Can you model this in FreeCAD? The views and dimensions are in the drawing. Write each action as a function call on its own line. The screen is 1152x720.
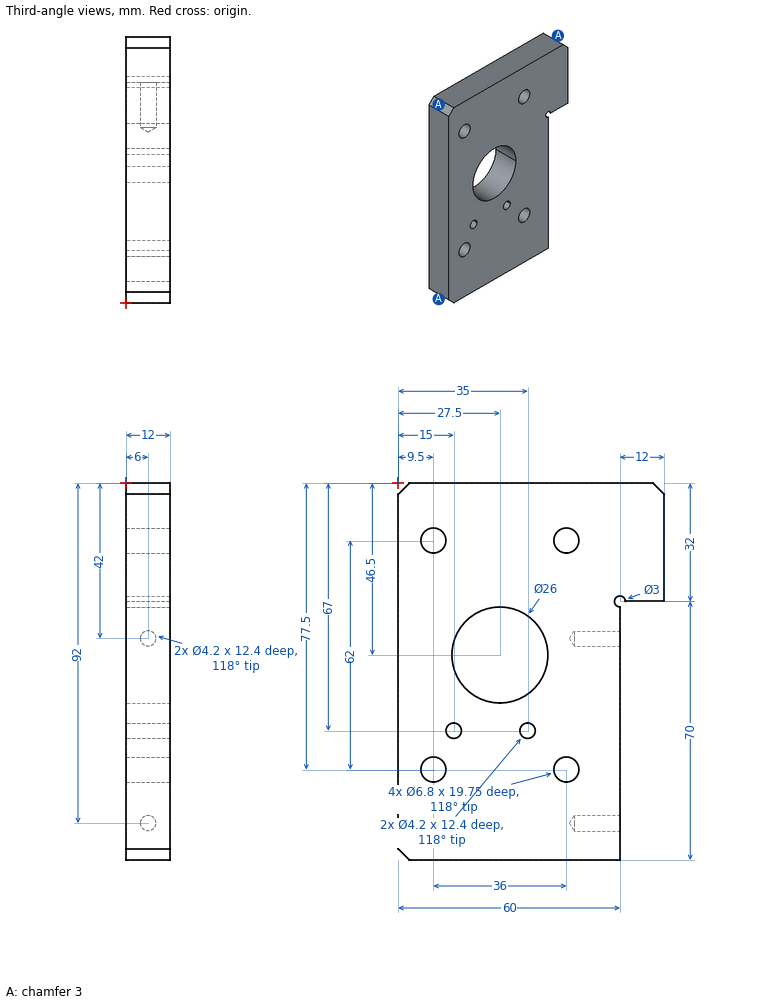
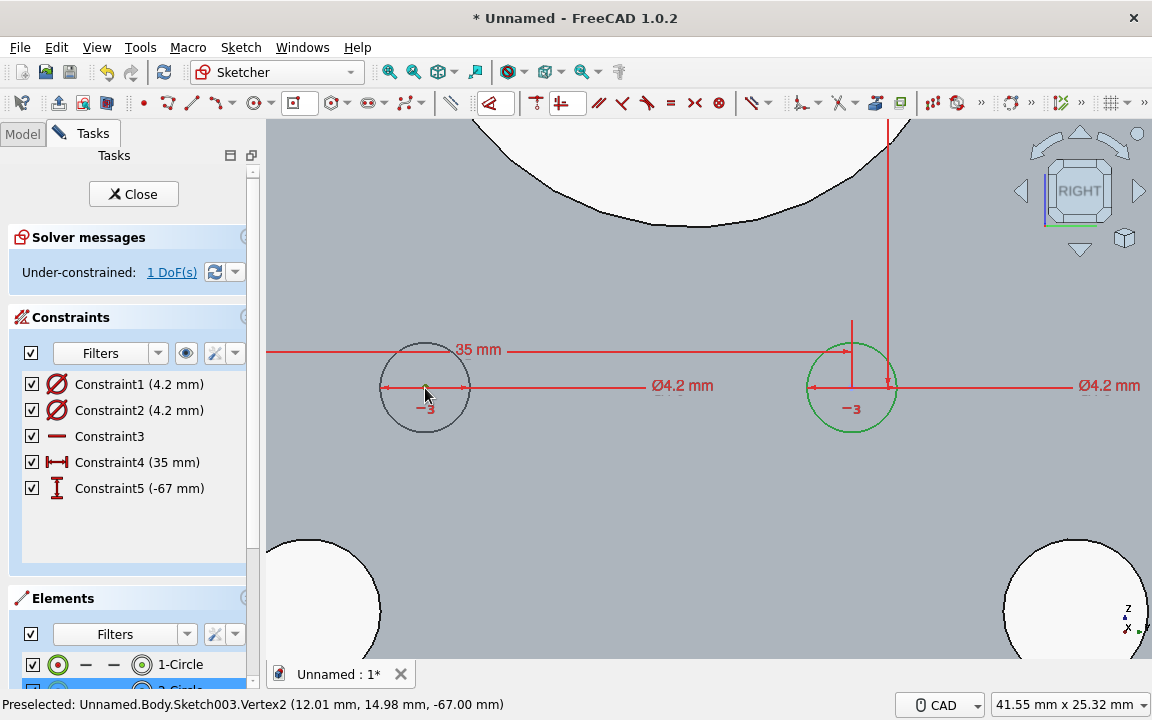
key(l)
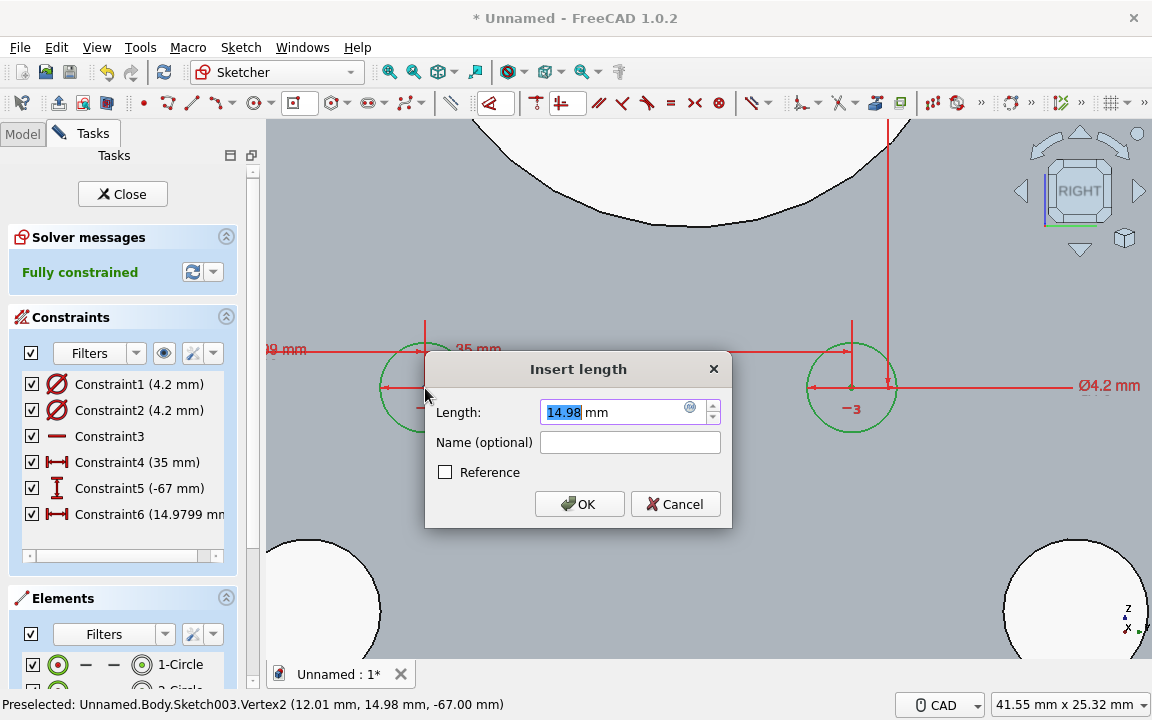
text(15)
key(Return)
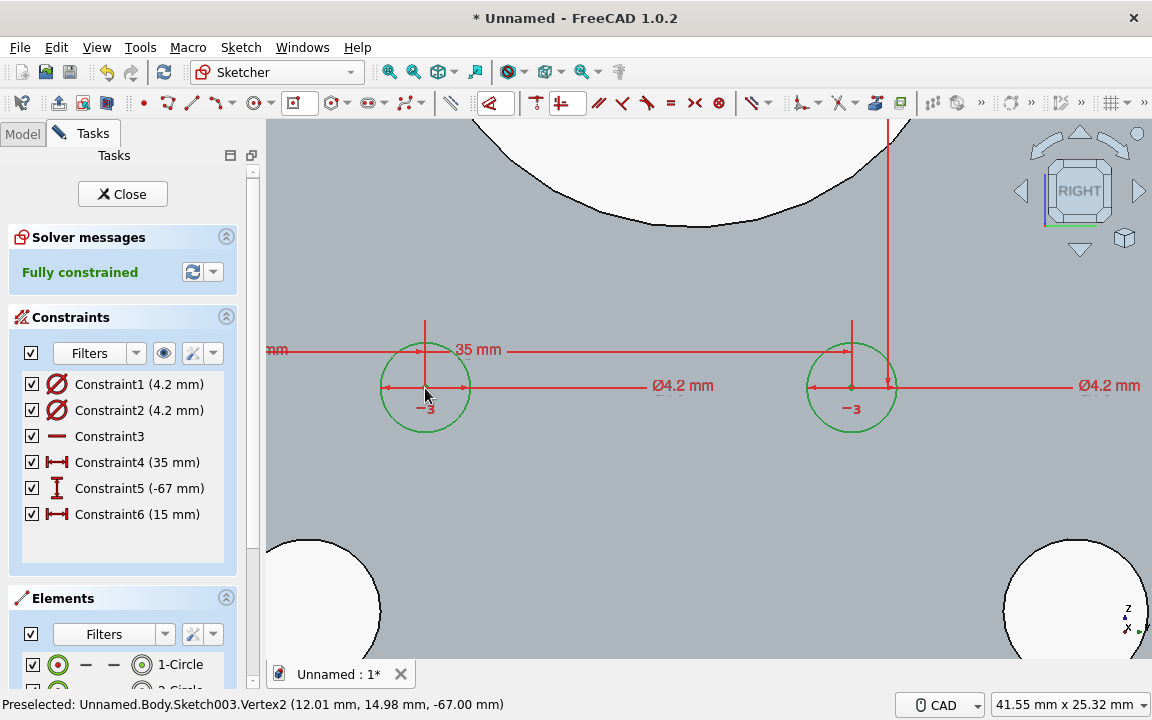
click(123, 194)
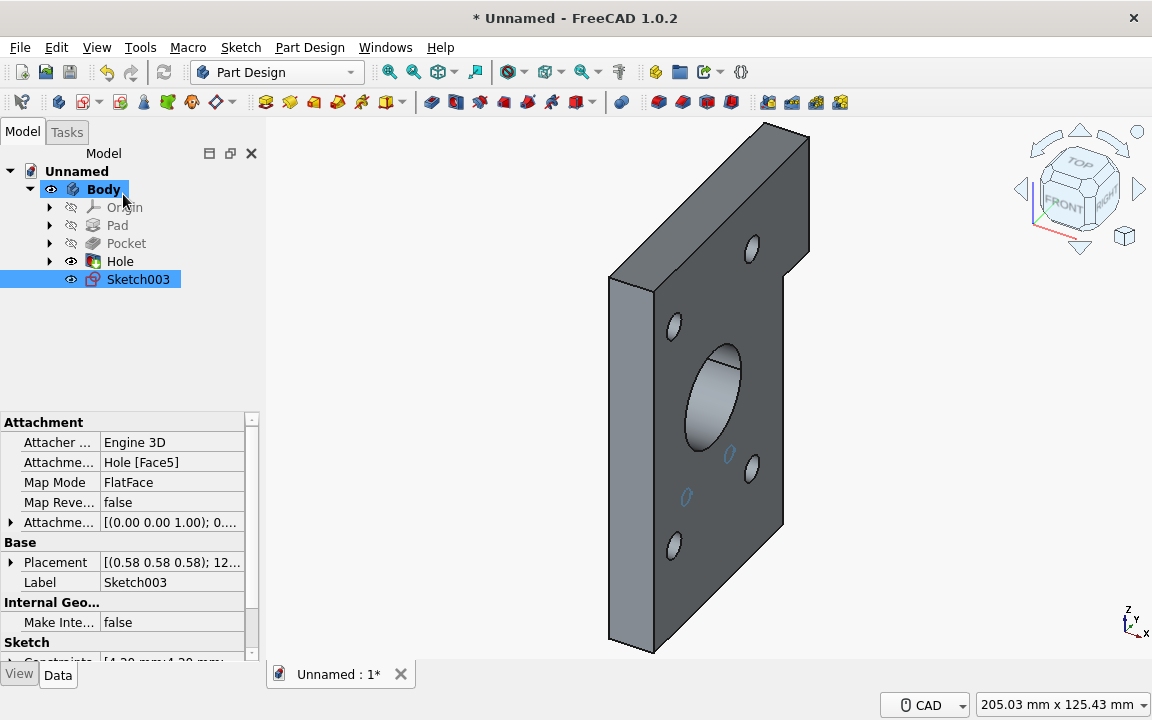
click(456, 102)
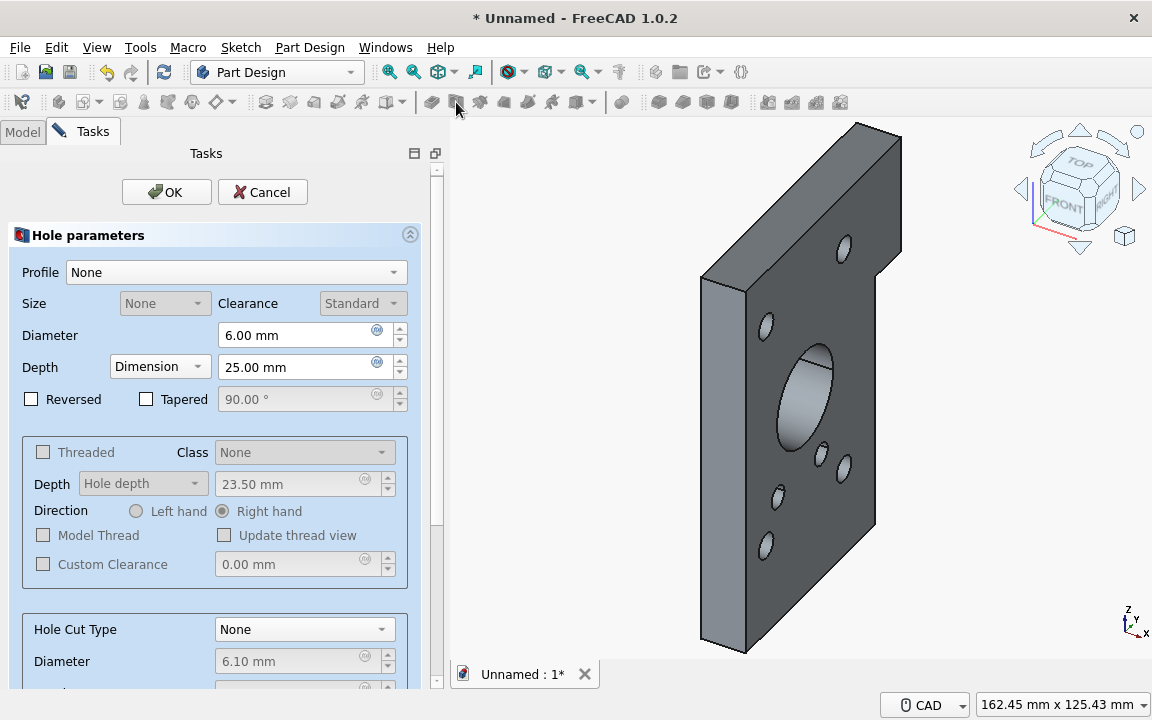
triple_click(305, 335)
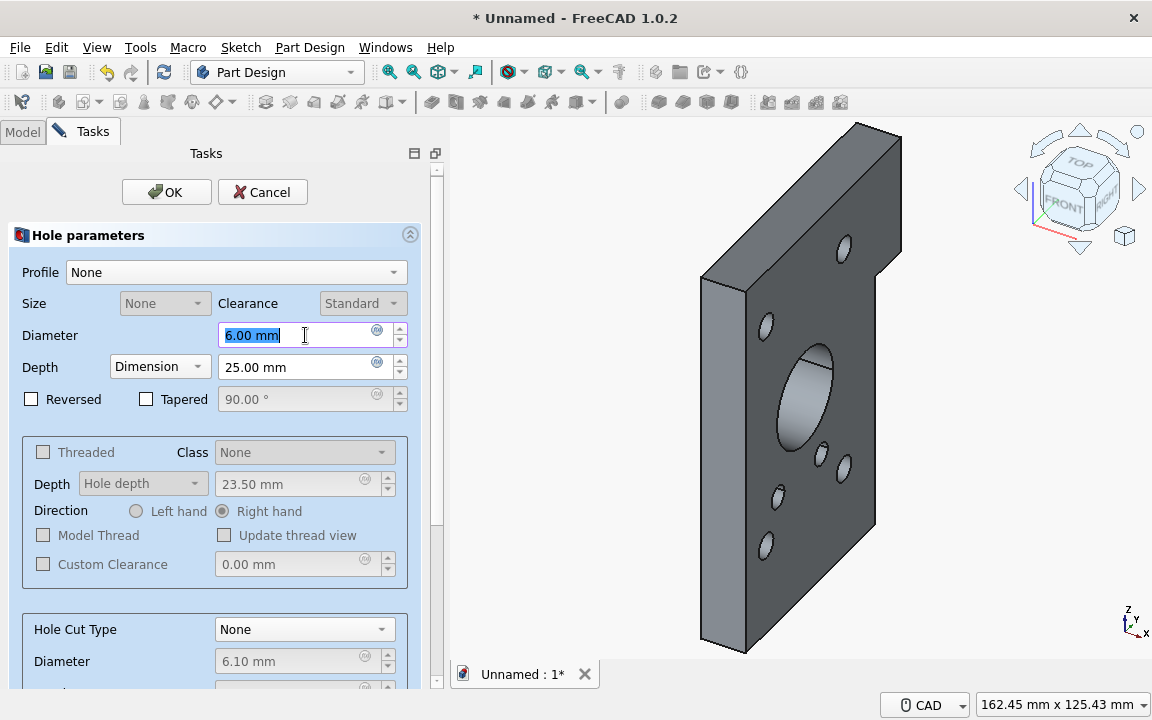
text(4.2)
key(Tab)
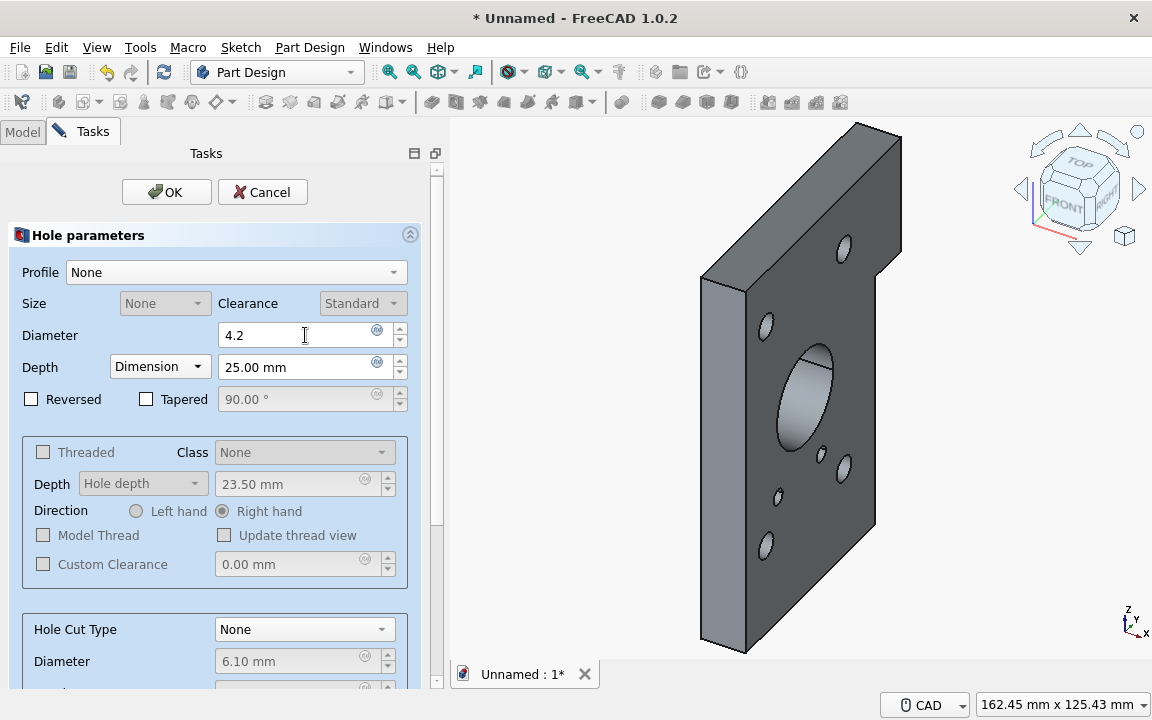
triple_click(305, 367)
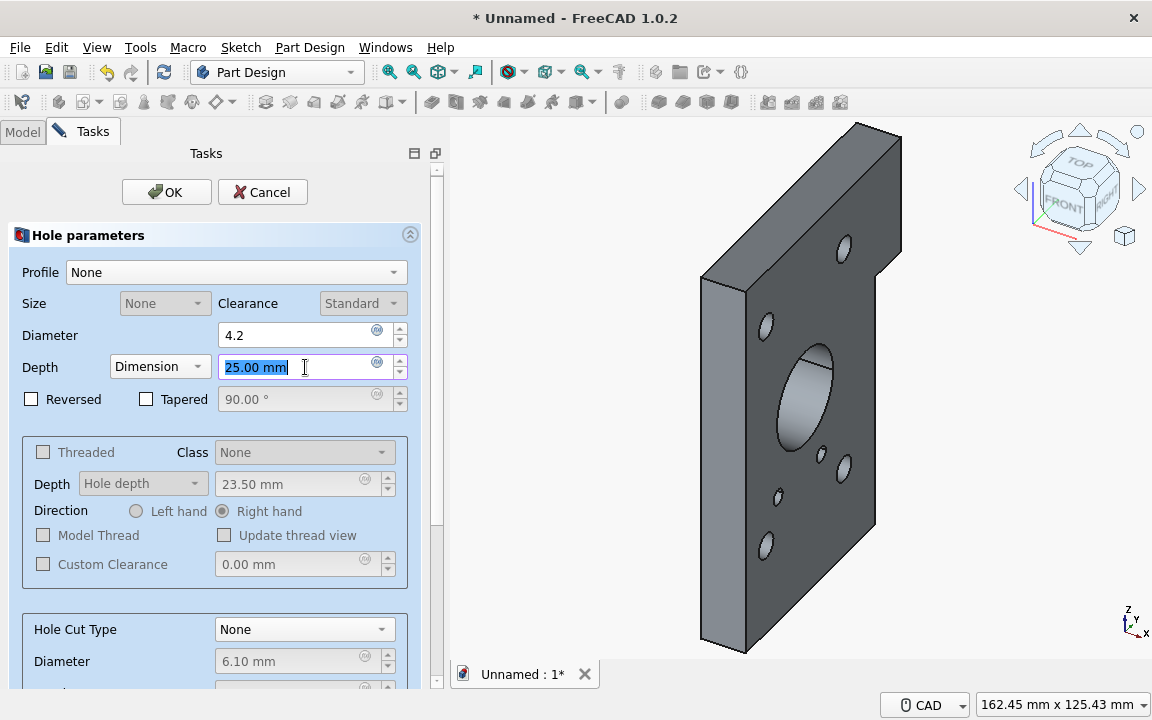
text(12.4)
key(Tab)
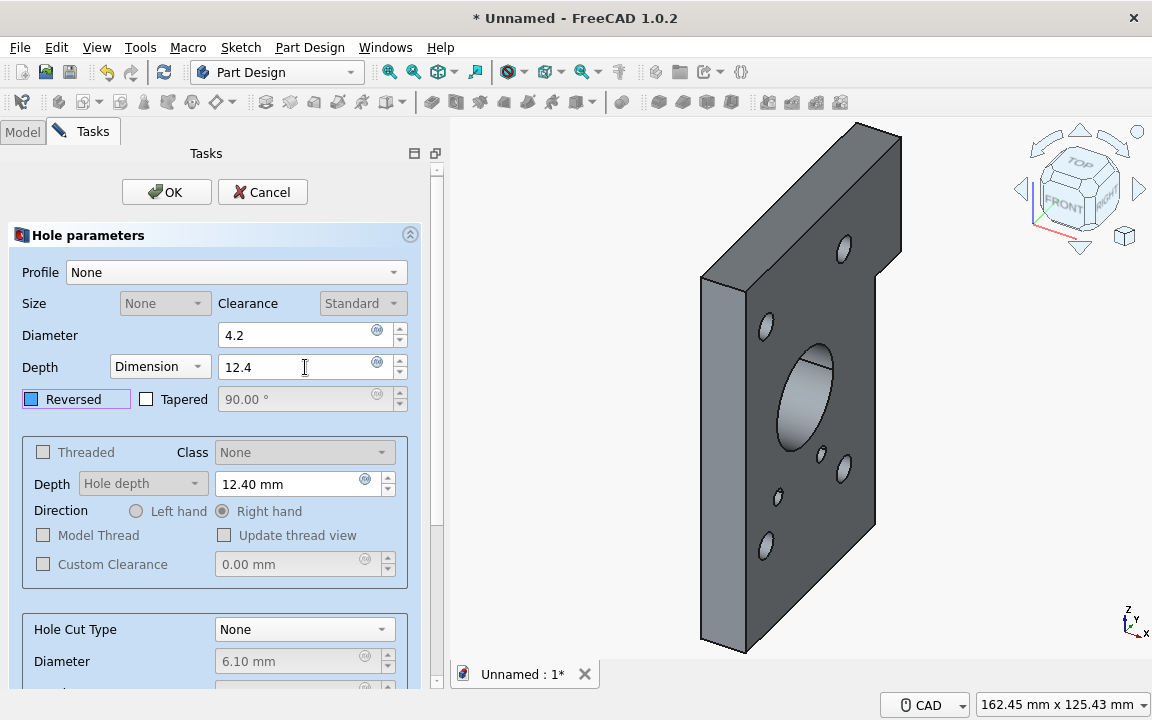
click(167, 192)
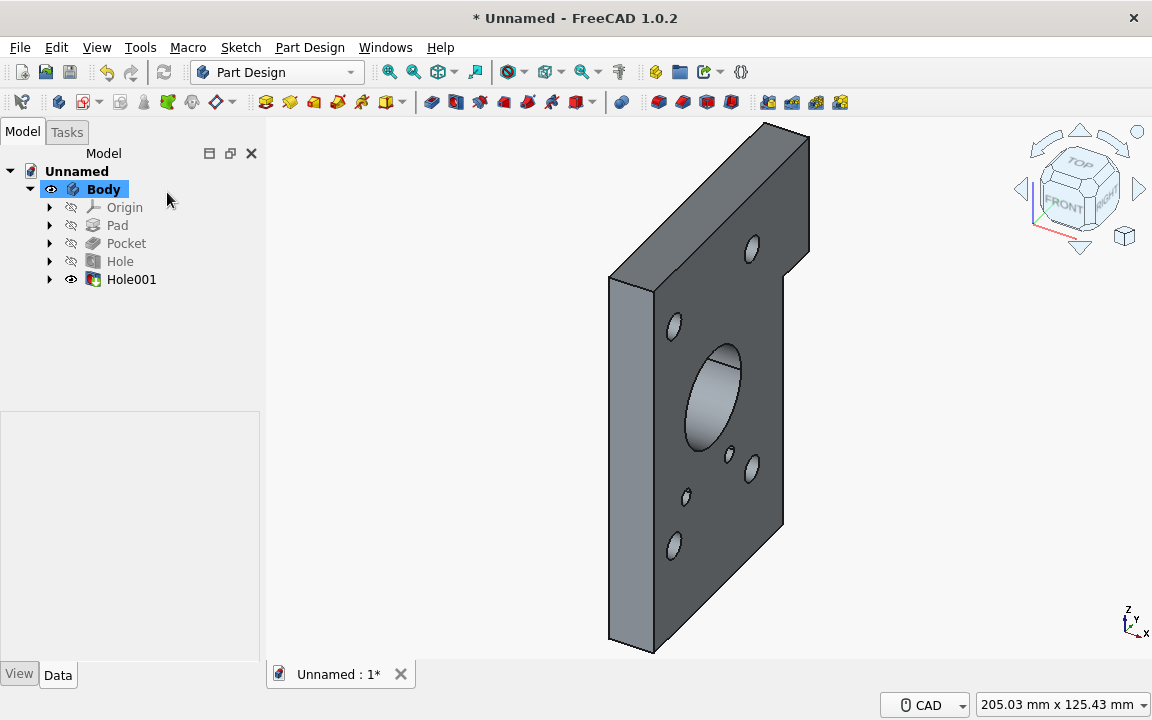
key(4)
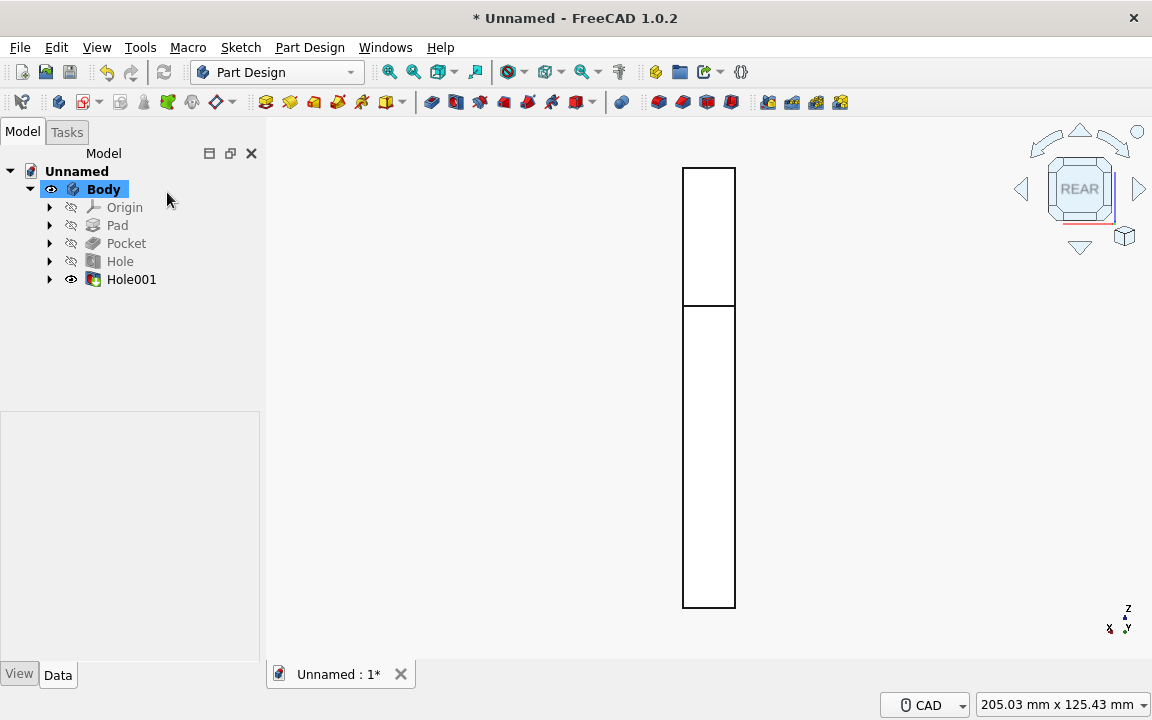
click(709, 543)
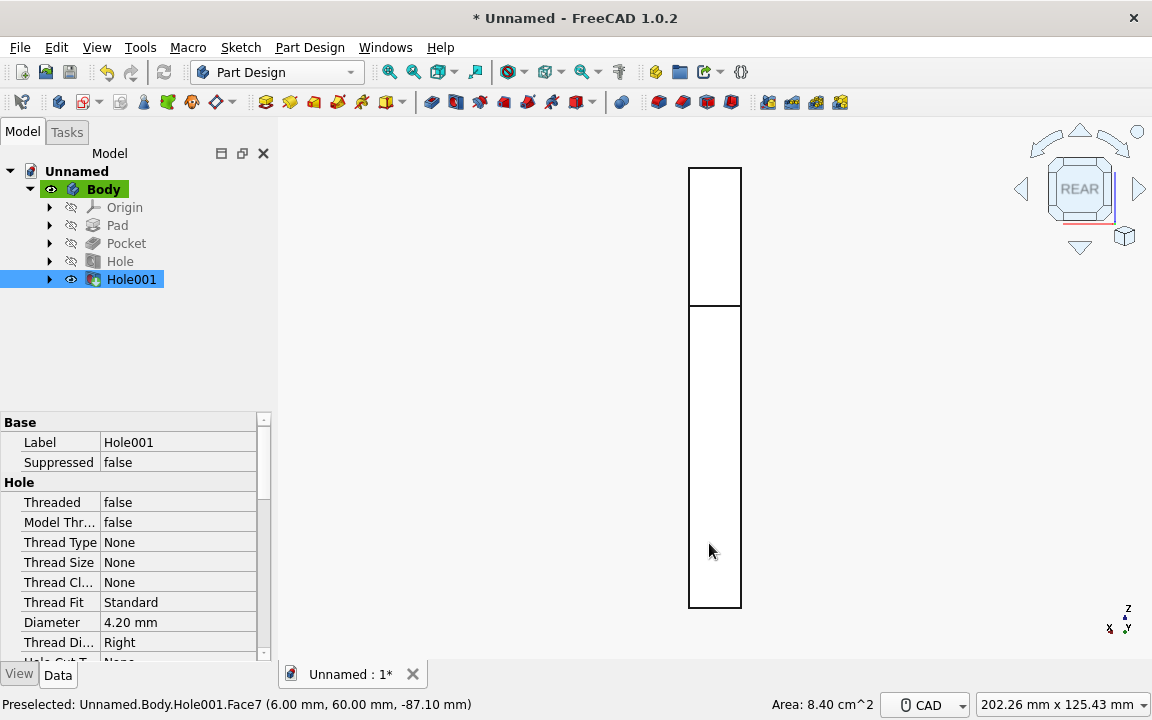
click(84, 102)